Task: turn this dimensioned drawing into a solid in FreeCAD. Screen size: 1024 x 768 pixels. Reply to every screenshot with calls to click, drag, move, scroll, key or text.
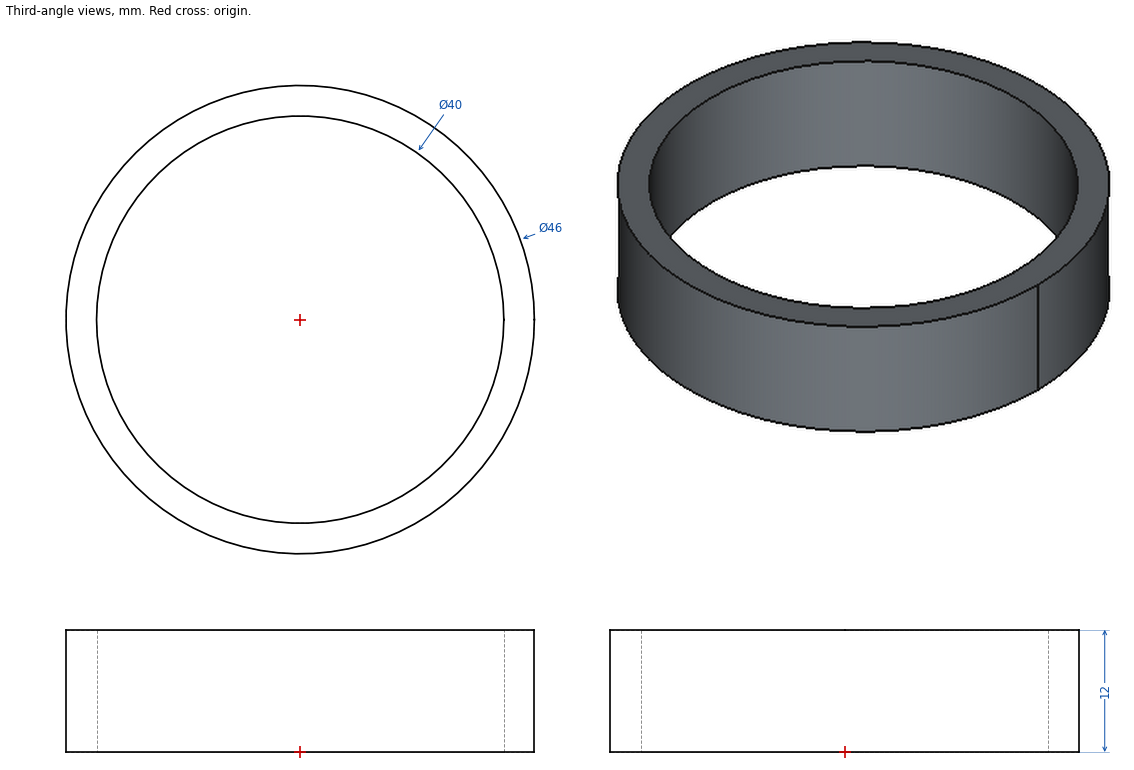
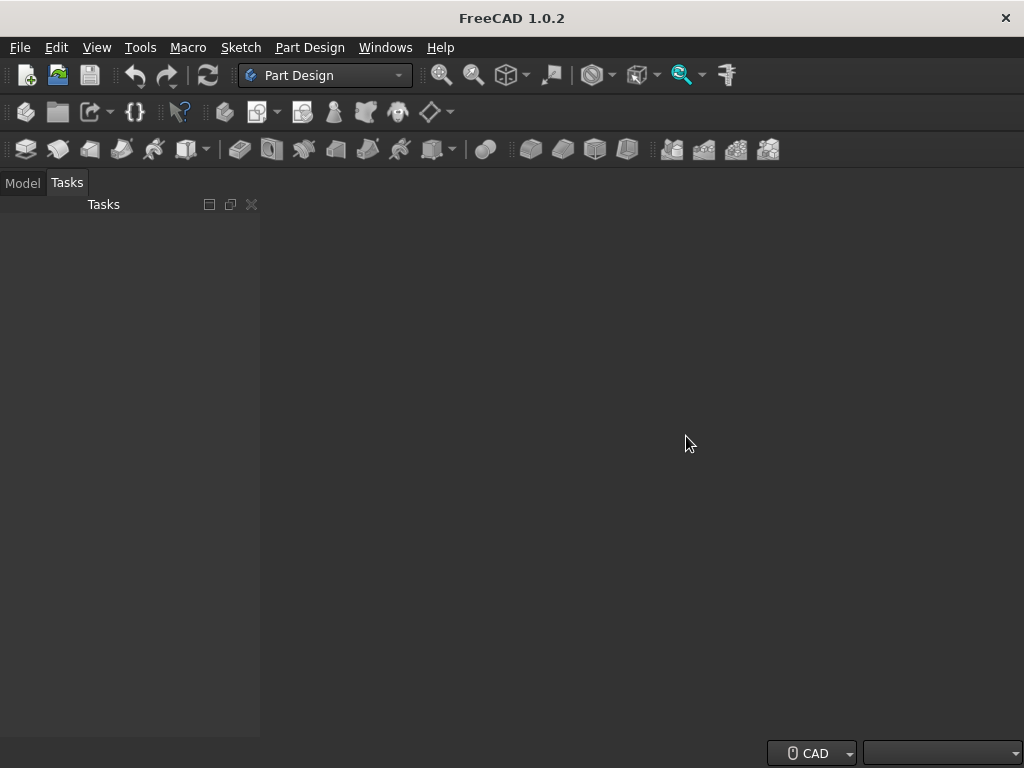
click(26, 76)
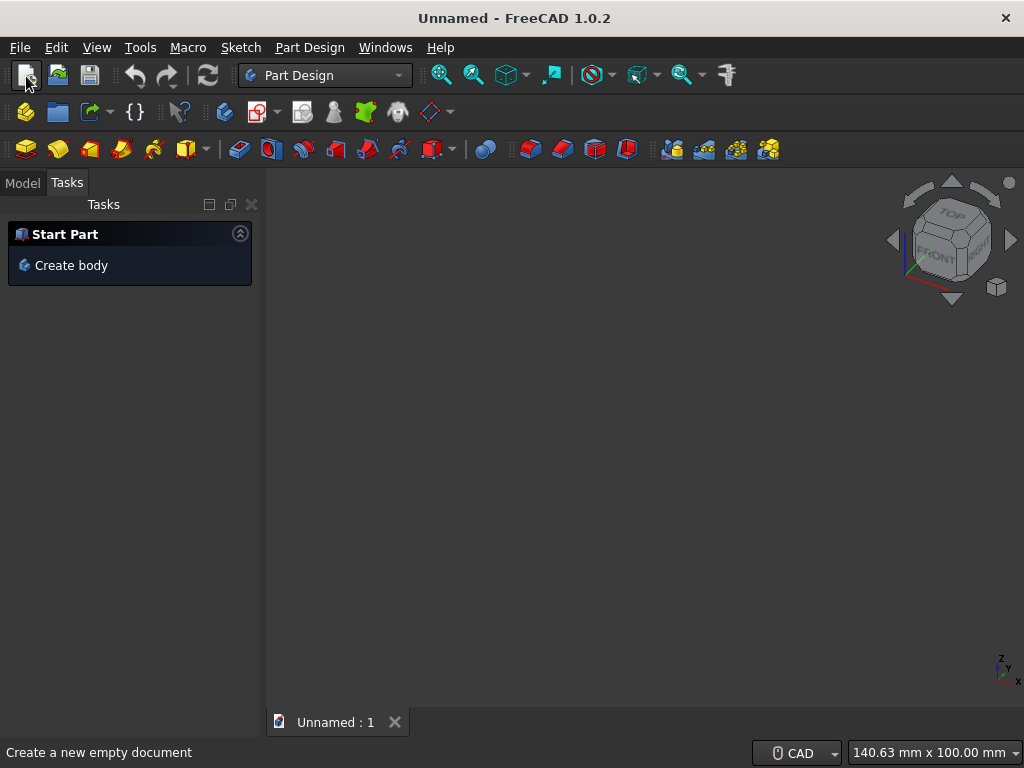
click(258, 112)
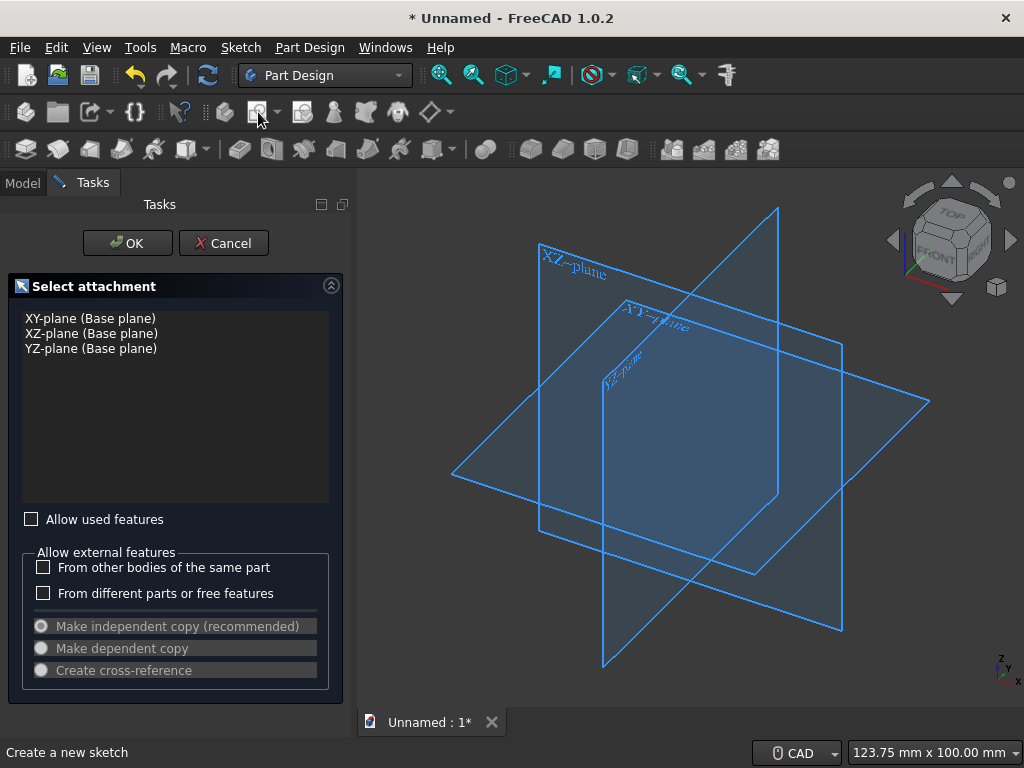
click(82, 318)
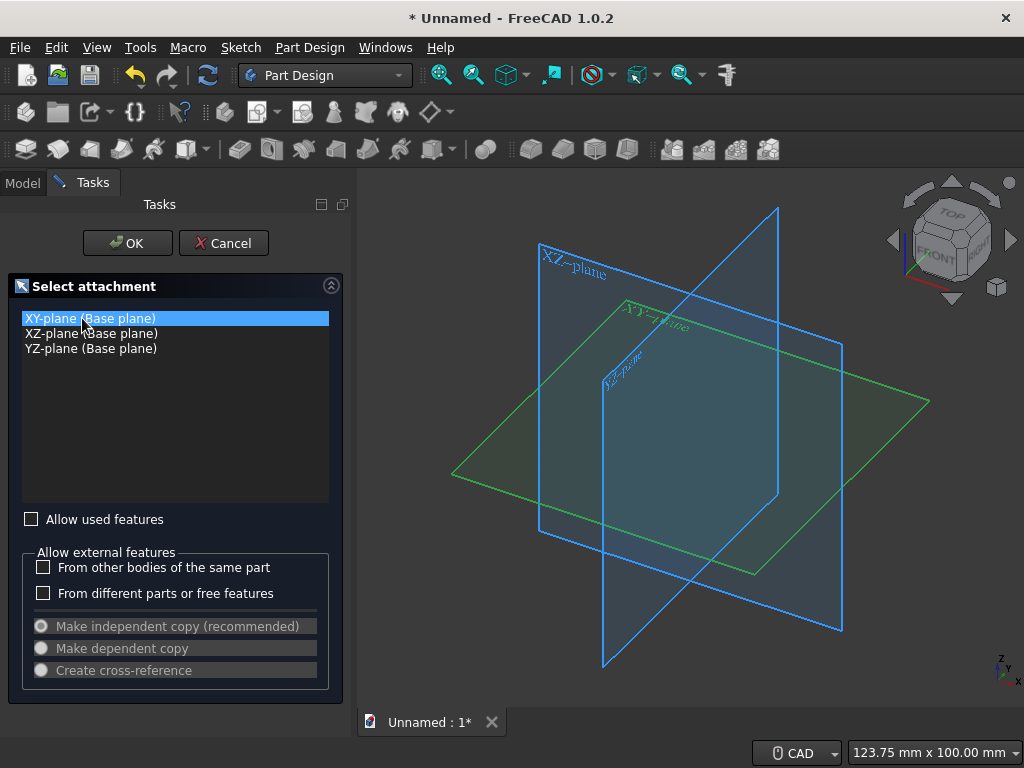
click(128, 243)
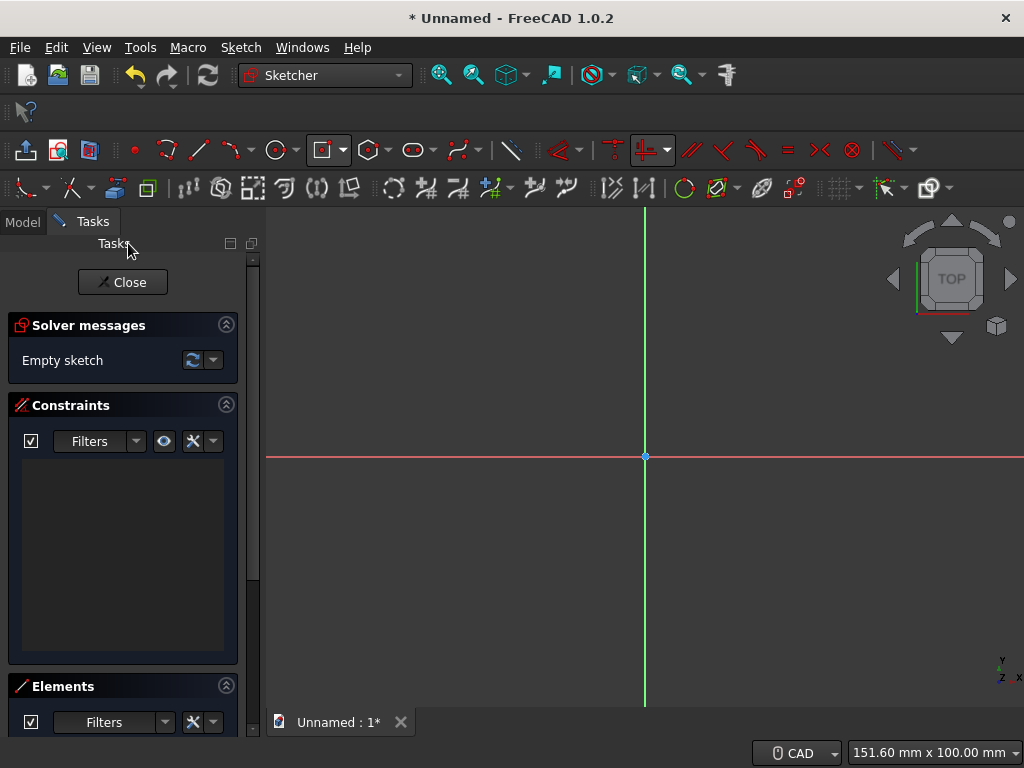
scroll(784, 457, up, 2)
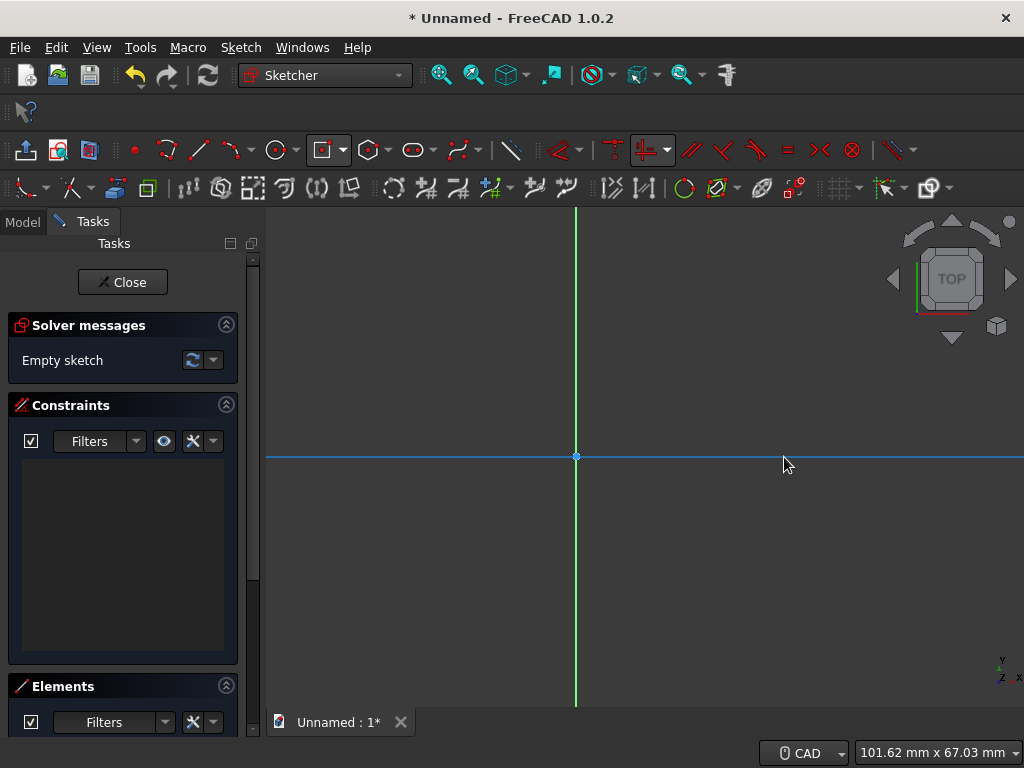
click(276, 150)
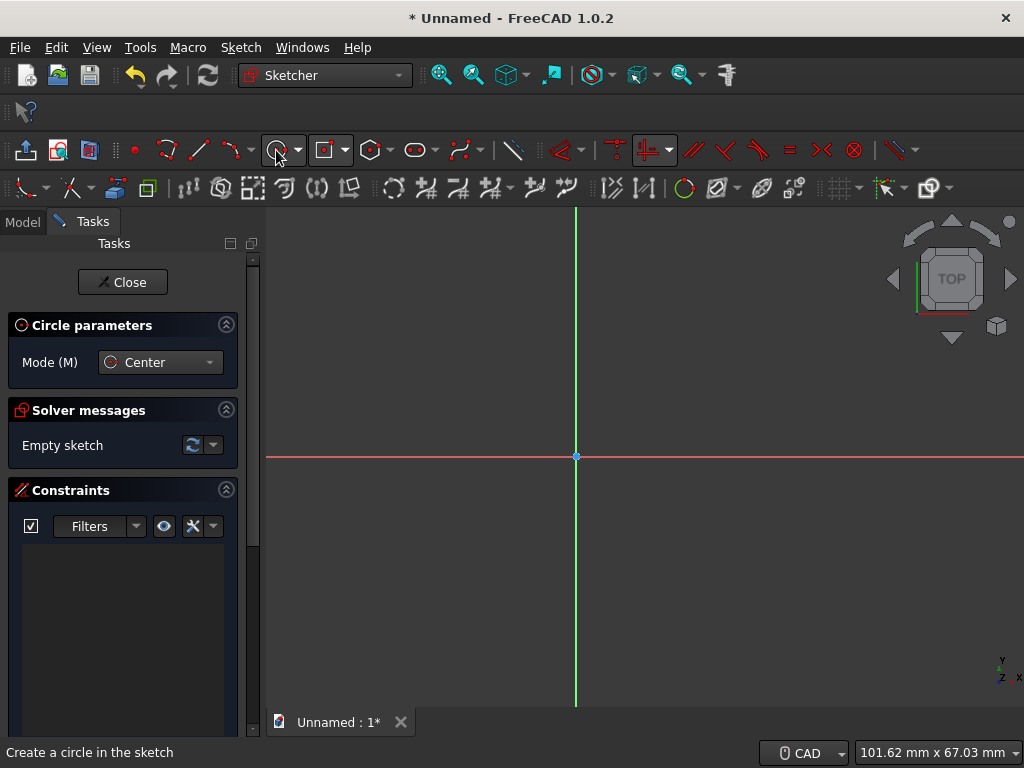
click(576, 457)
move(698, 335)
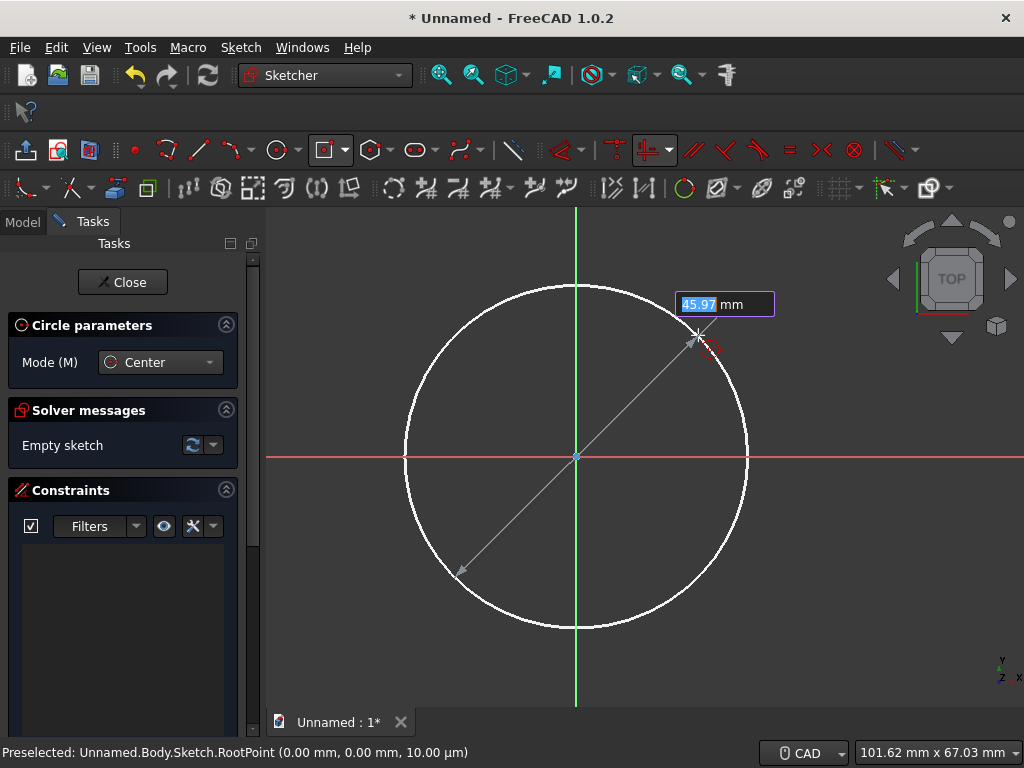
text(46)
key(Return)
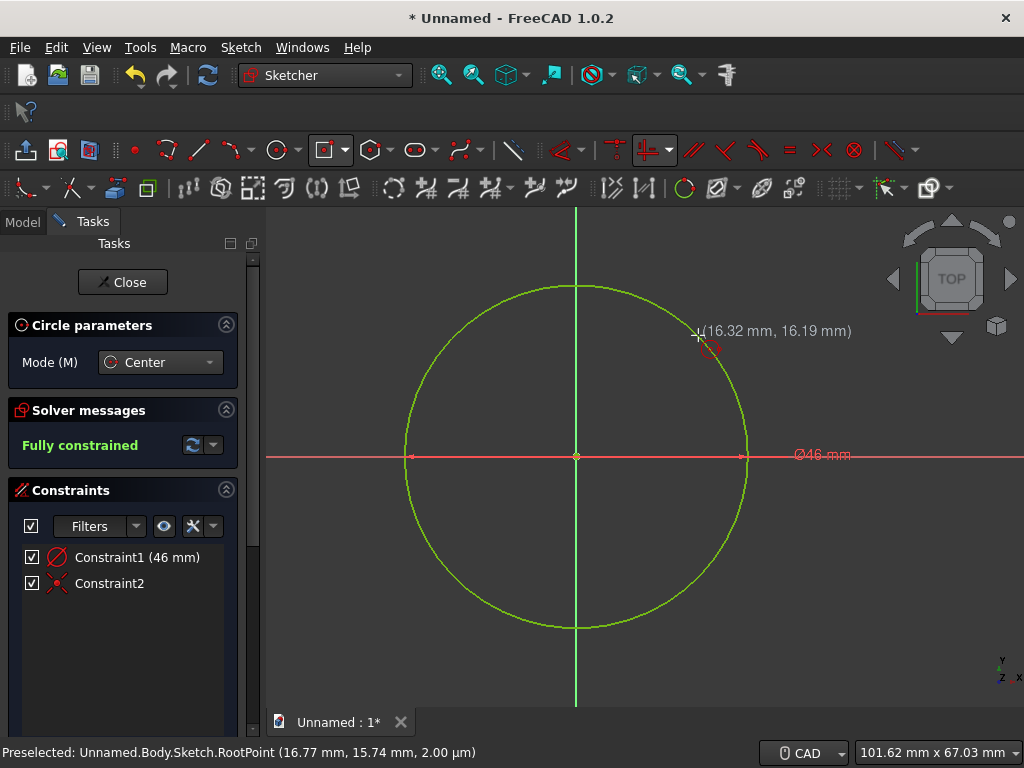
click(576, 457)
move(682, 351)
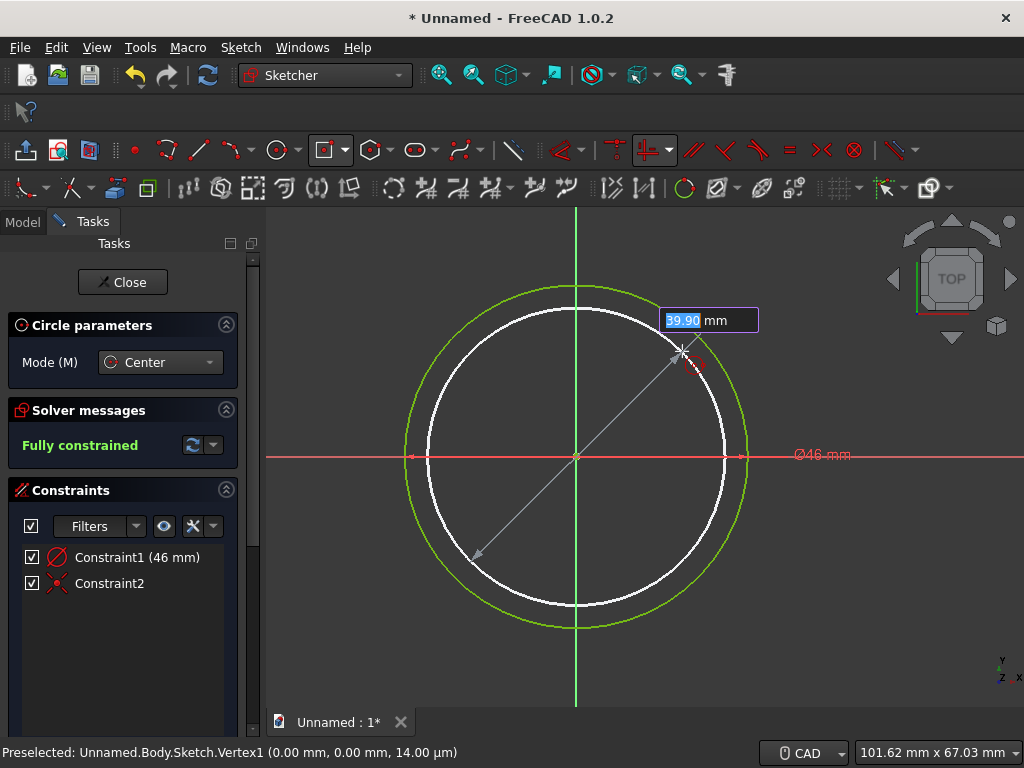
text(40)
key(Return)
key(Escape)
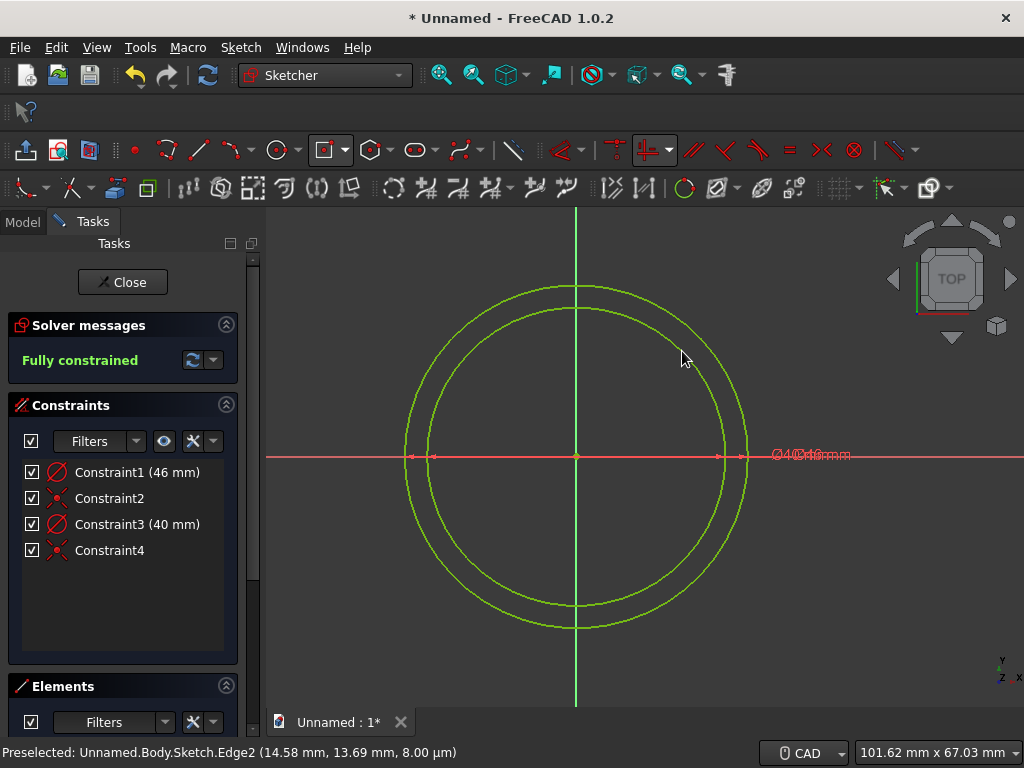
click(123, 282)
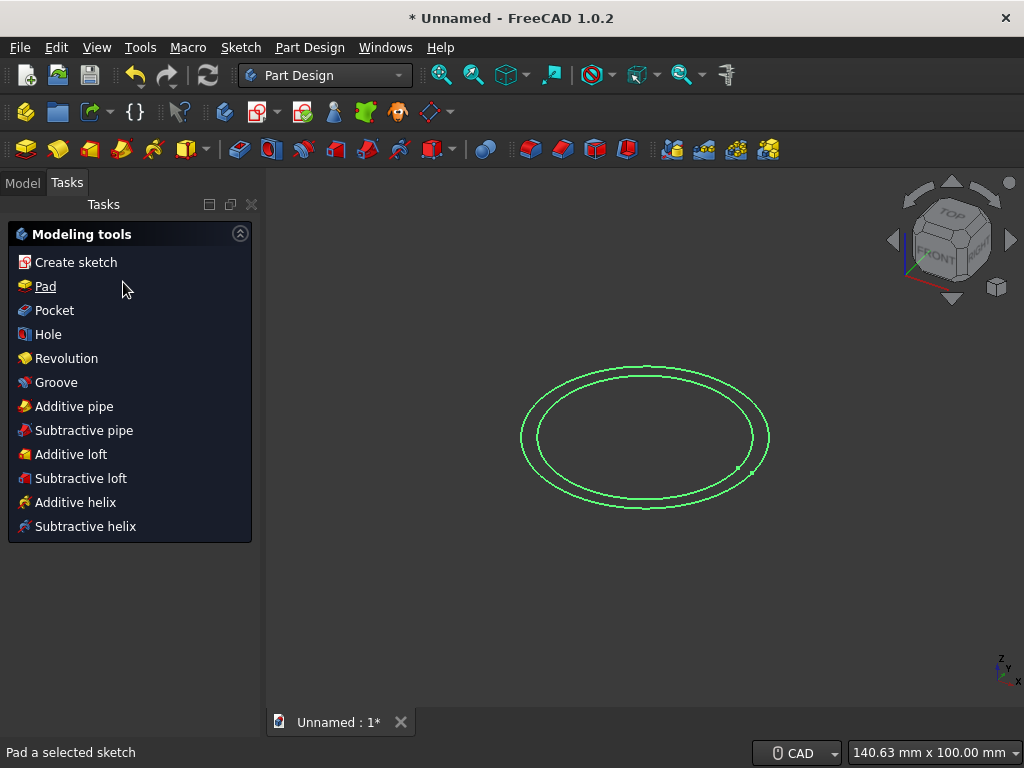
click(26, 150)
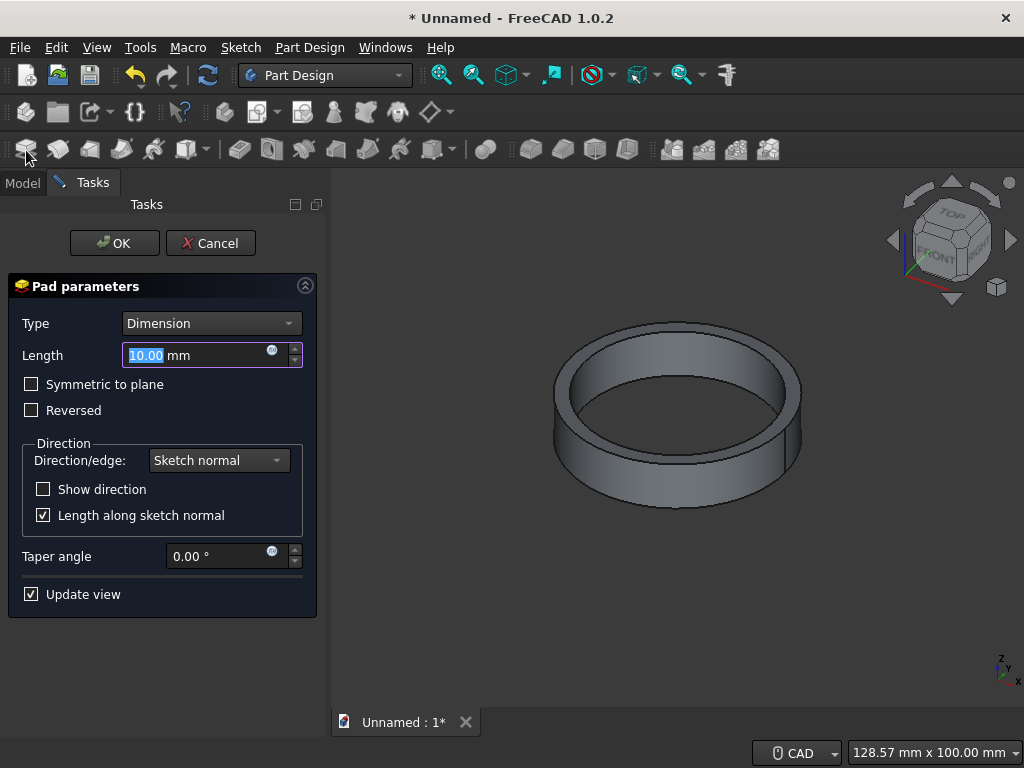
text(12)
key(Tab)